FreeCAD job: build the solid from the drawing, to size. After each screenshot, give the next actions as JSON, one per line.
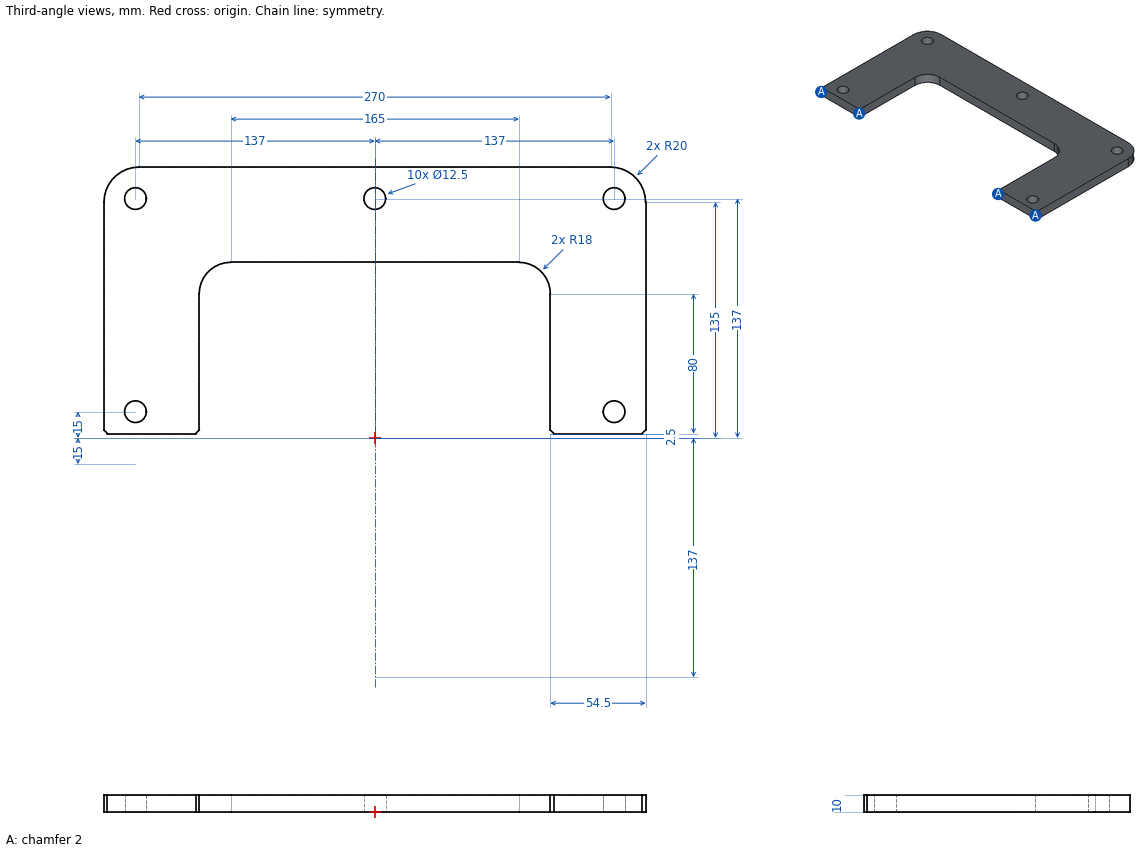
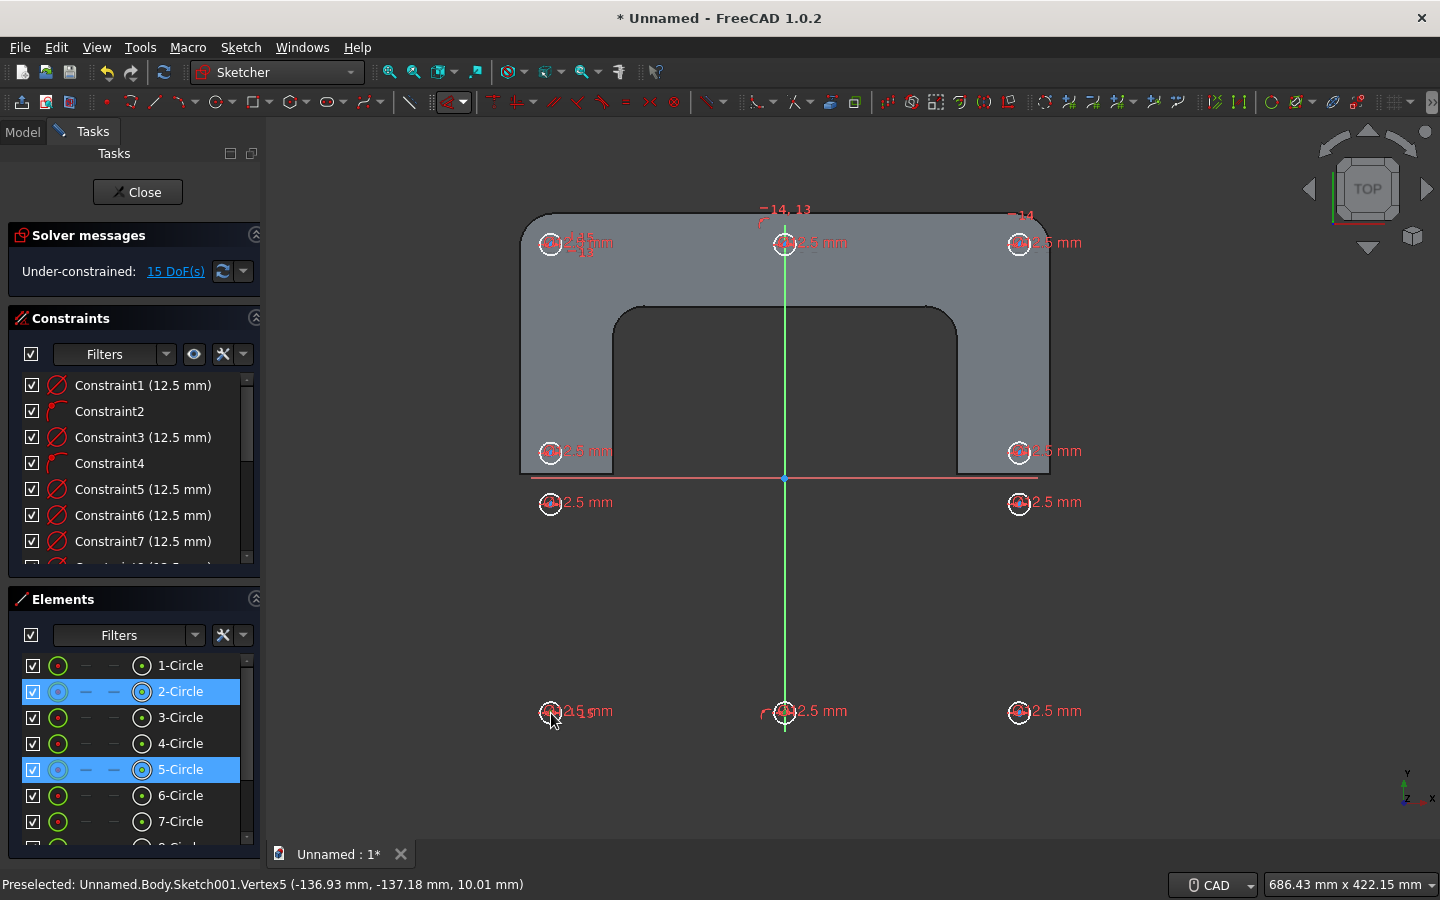
{"action": "key", "text": "h"}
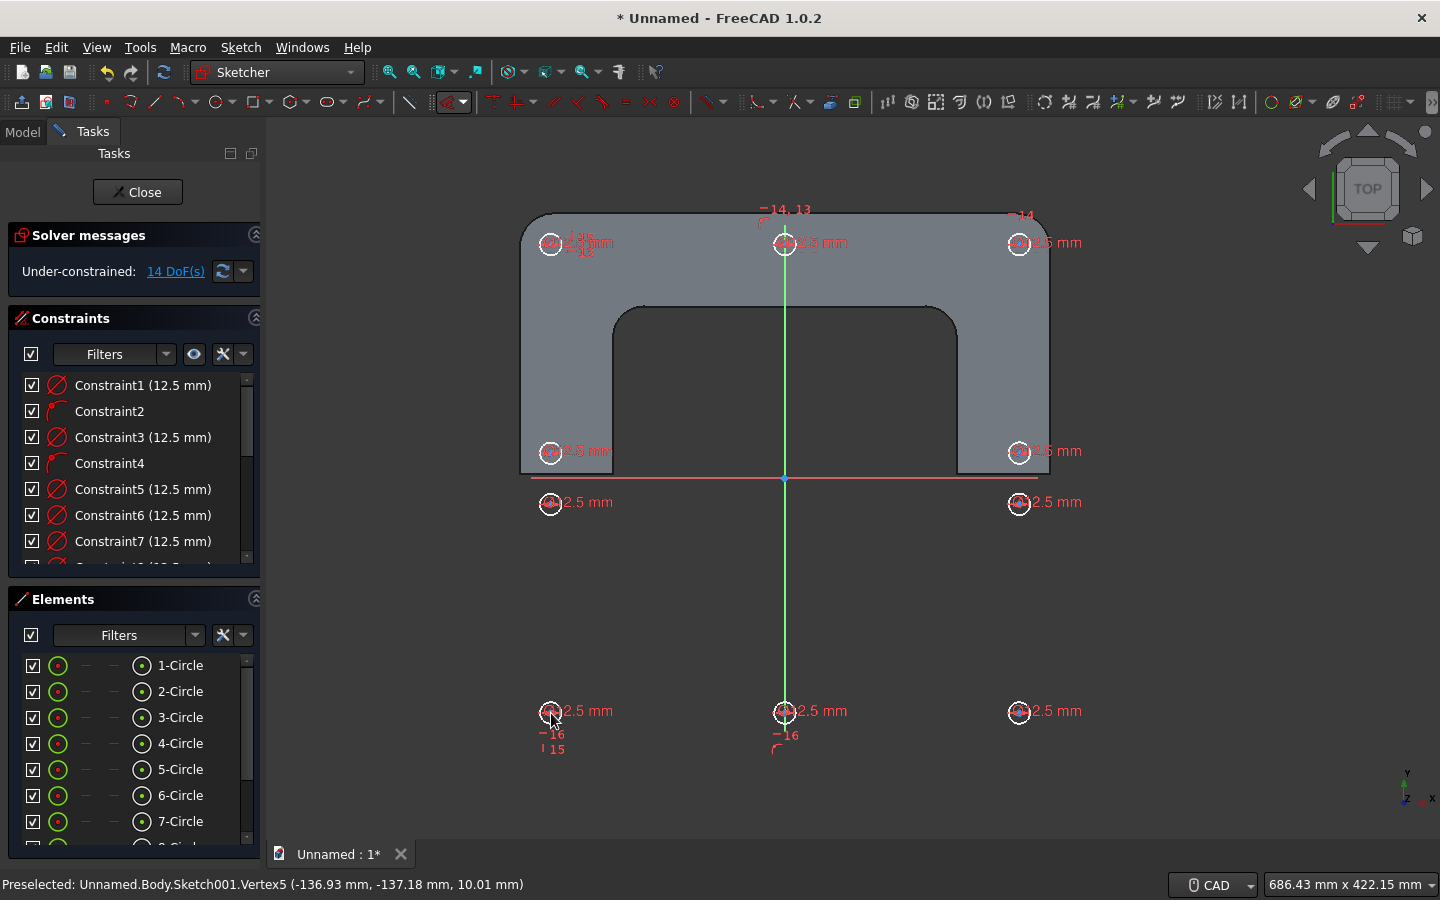
{"action": "left_click", "coordinate": [1019, 245]}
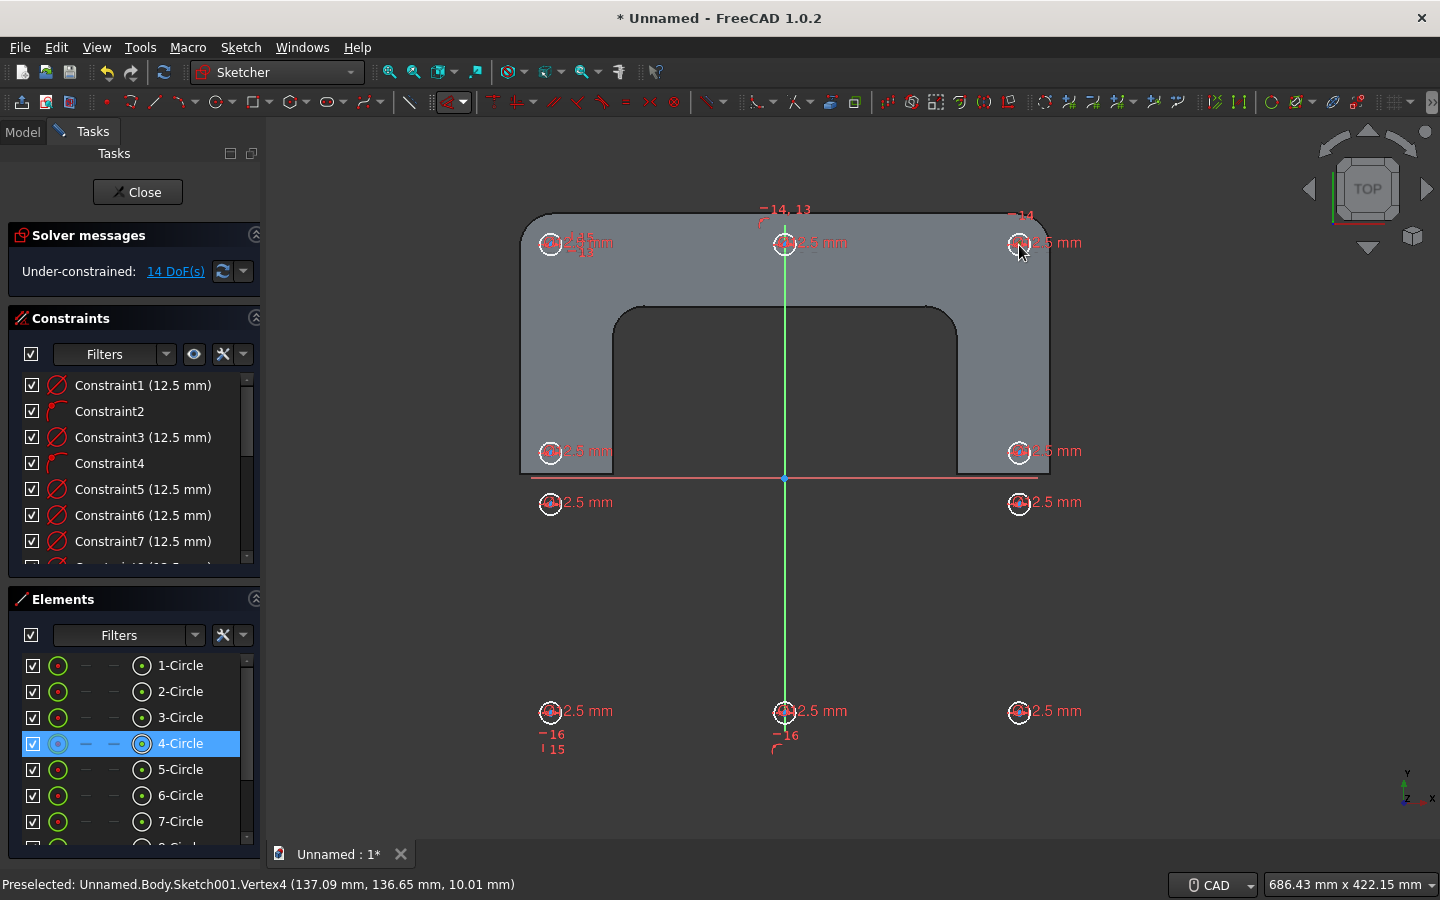
{"action": "left_click", "coordinate": [1019, 713]}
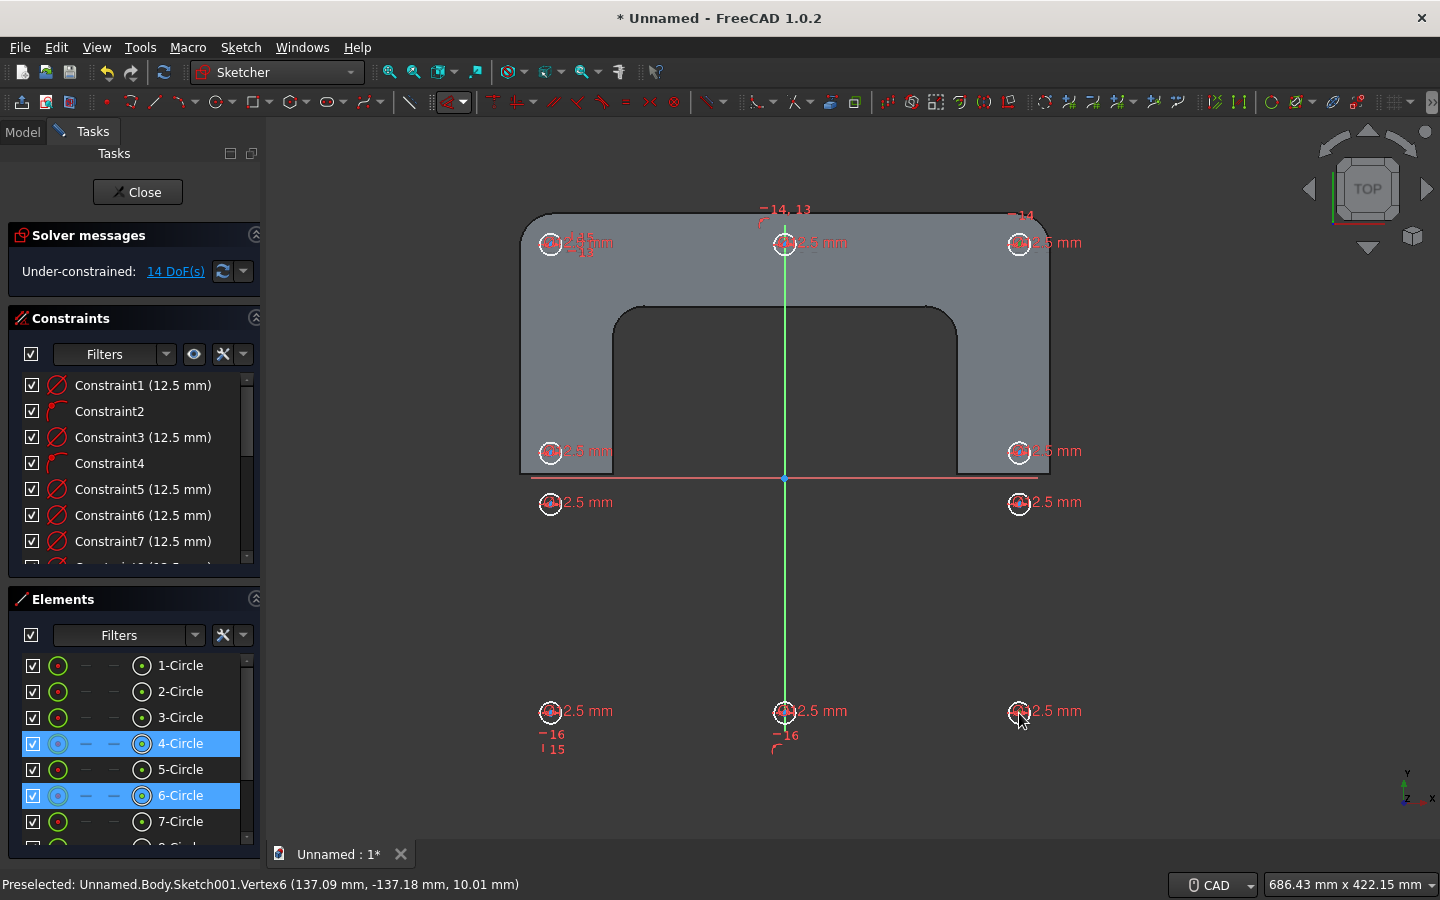
{"action": "key", "text": "v"}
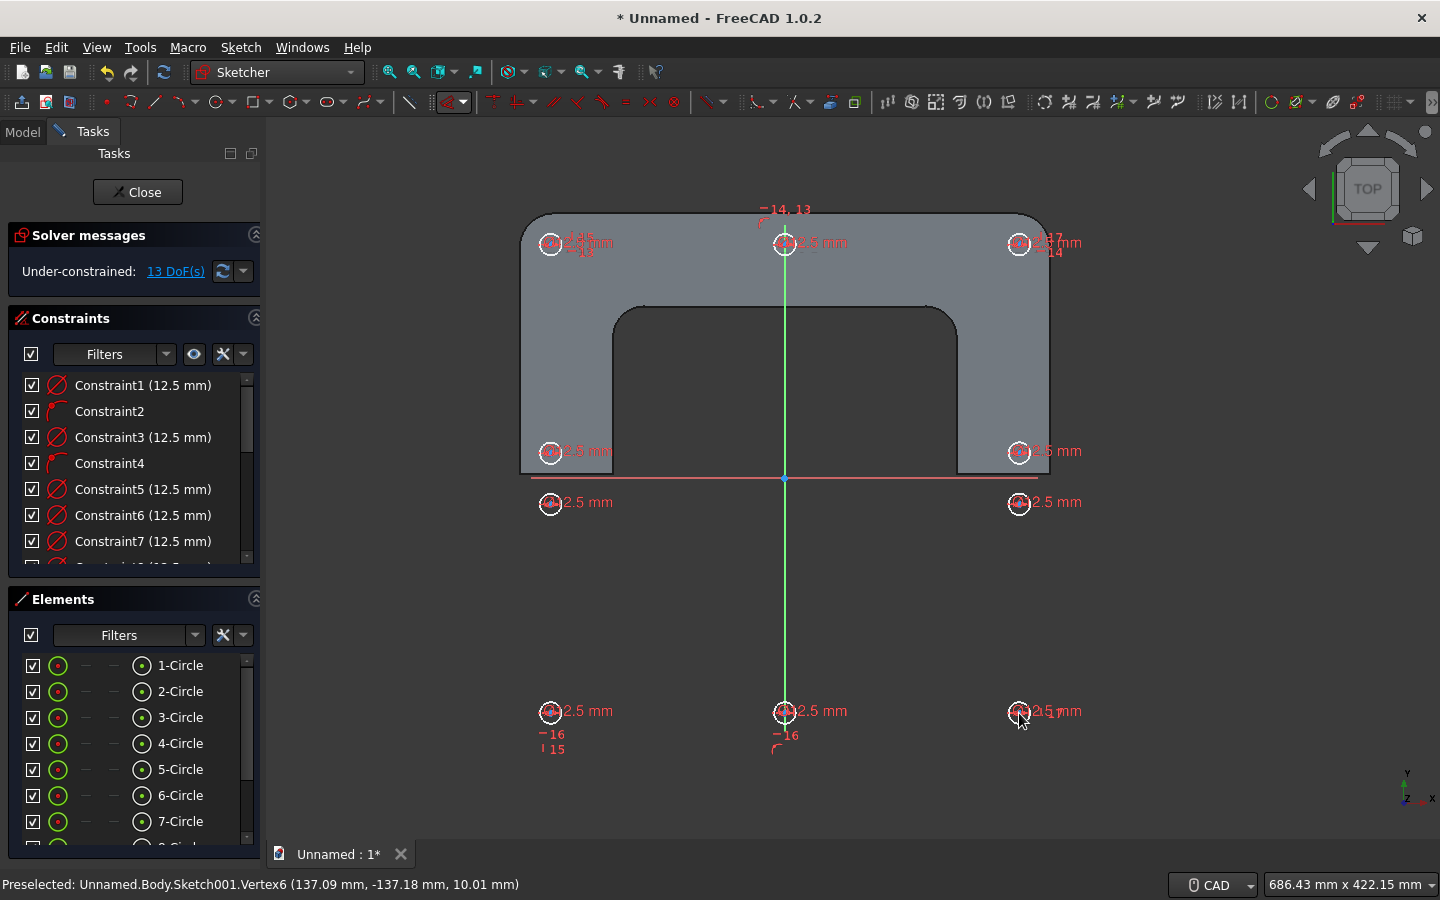
{"action": "left_click", "coordinate": [785, 713]}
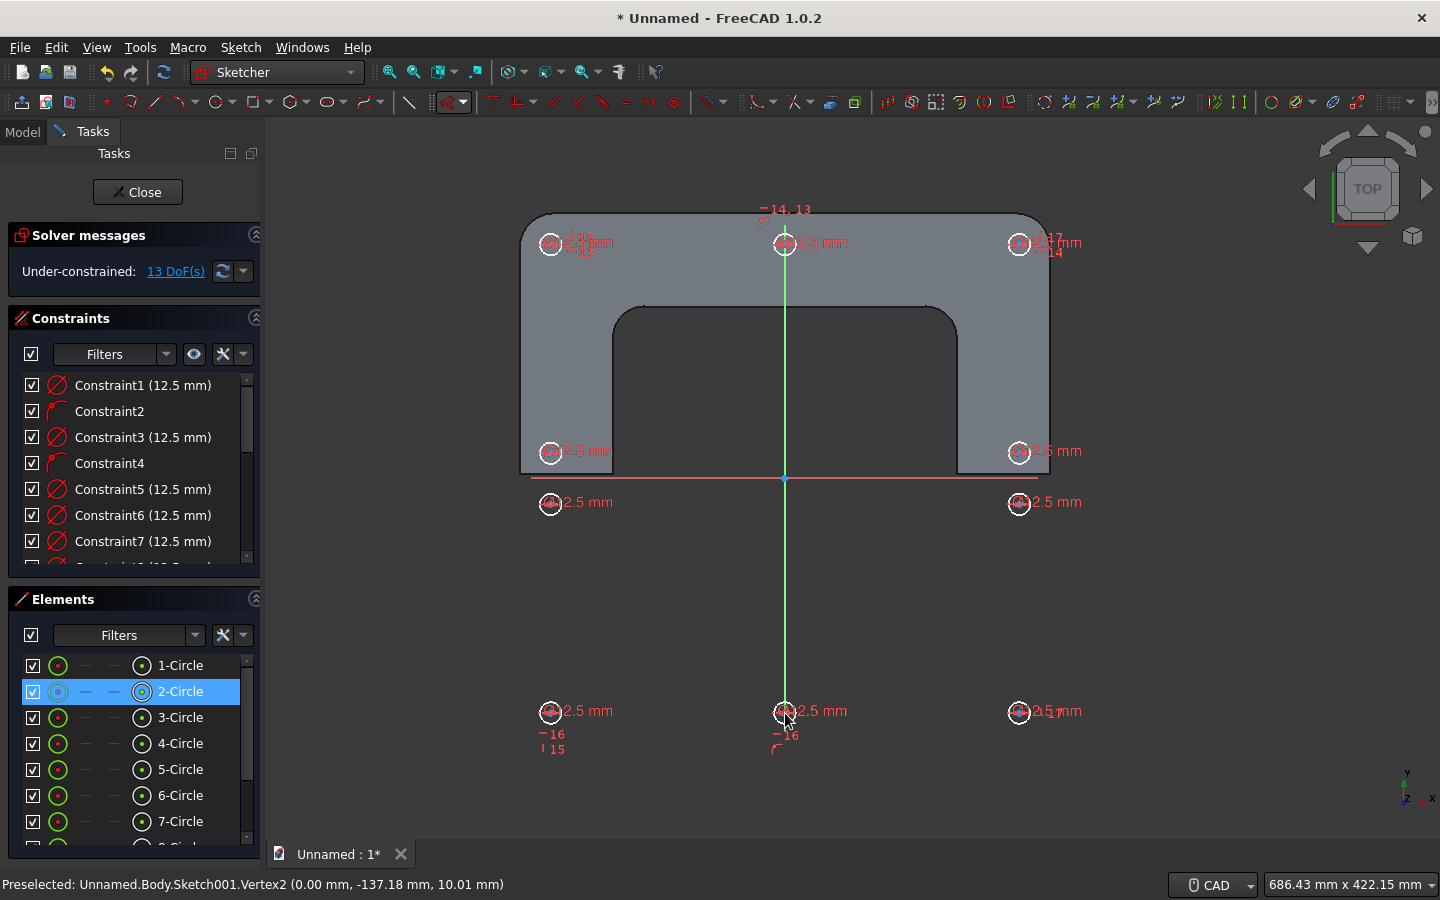
{"action": "left_click", "coordinate": [1019, 713]}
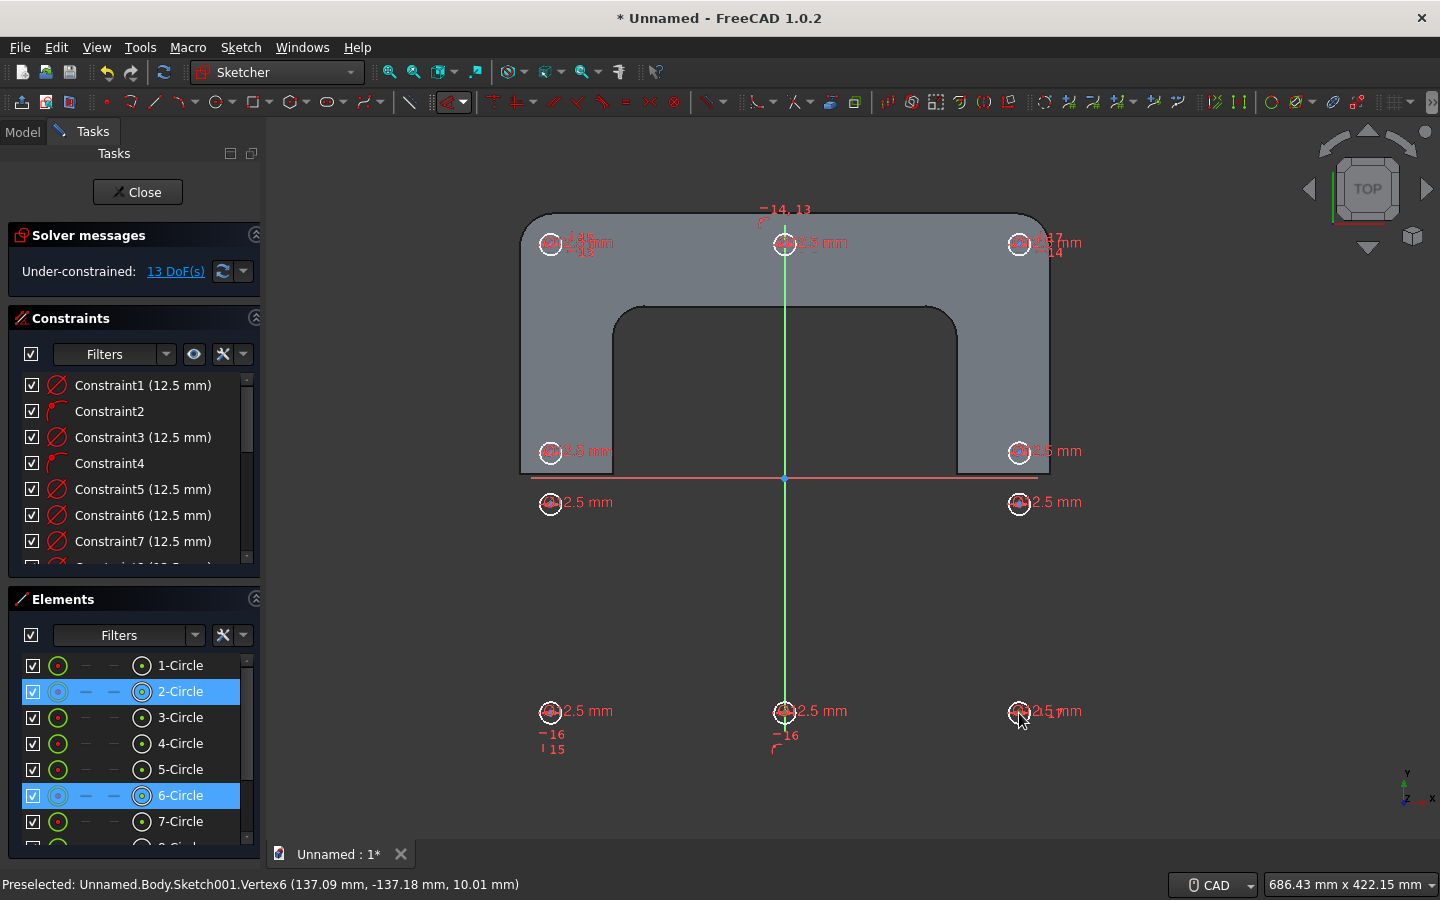
{"action": "left_click", "coordinate": [536, 102]}